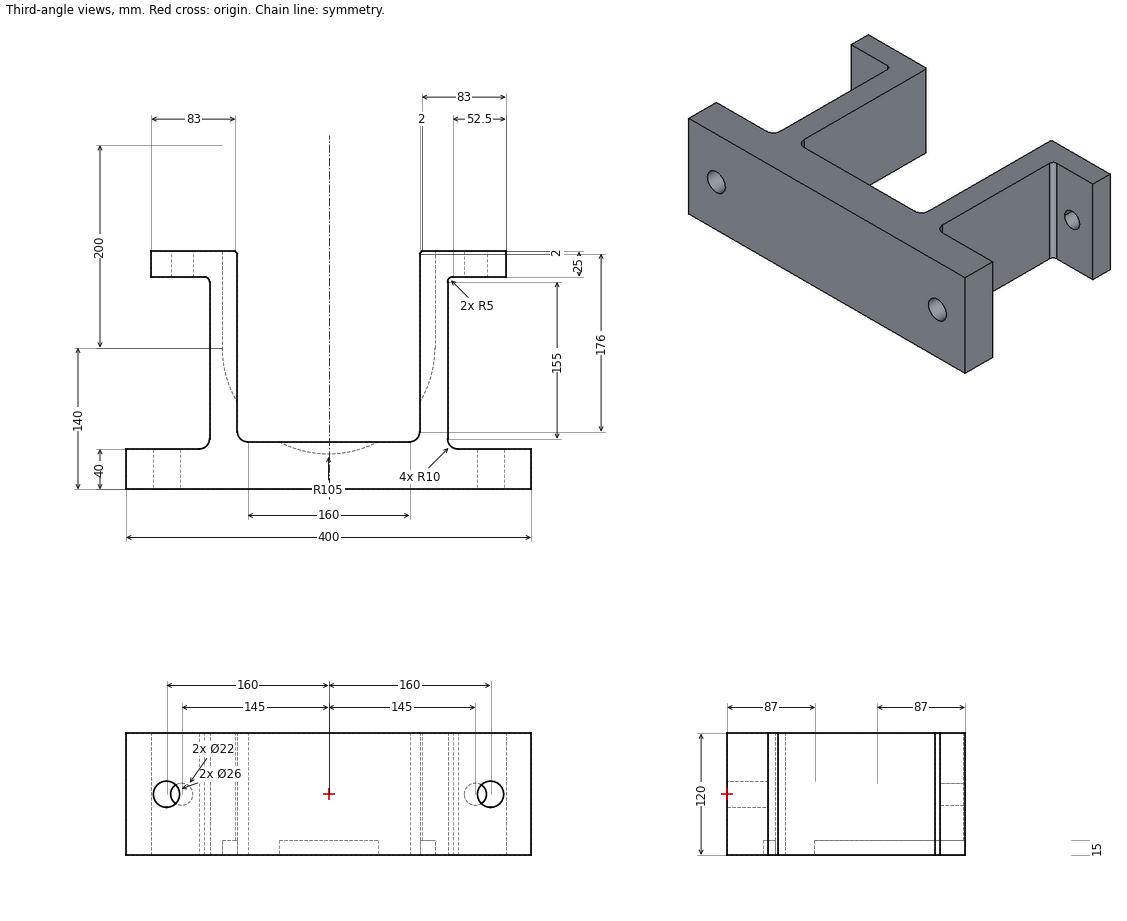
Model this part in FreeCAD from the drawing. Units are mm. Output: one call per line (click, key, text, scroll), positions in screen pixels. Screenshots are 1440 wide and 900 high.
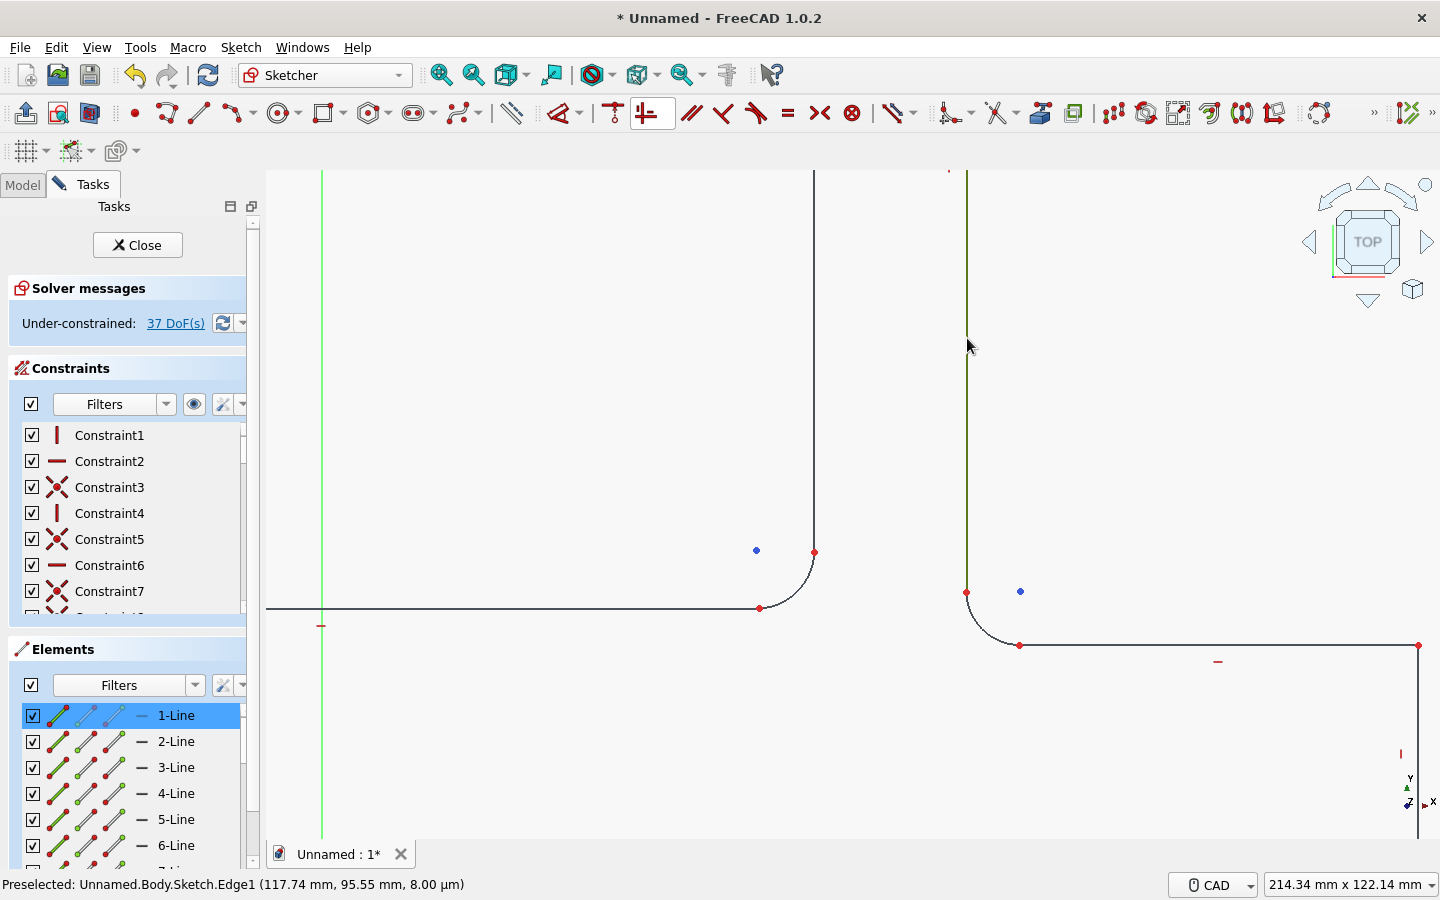
scroll(984, 628, down, 6)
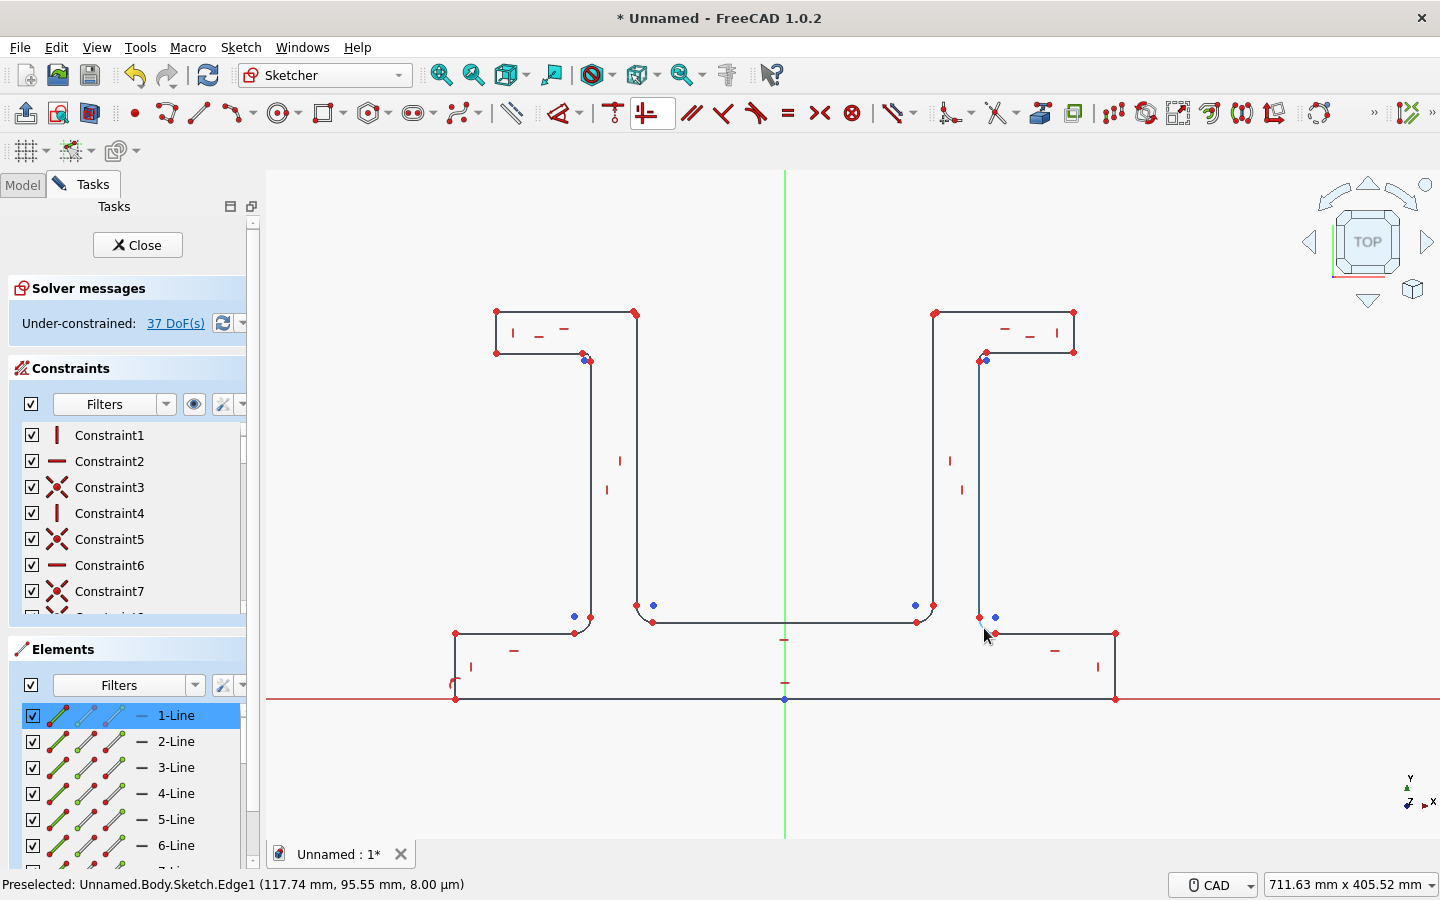
scroll(983, 354, up, 7)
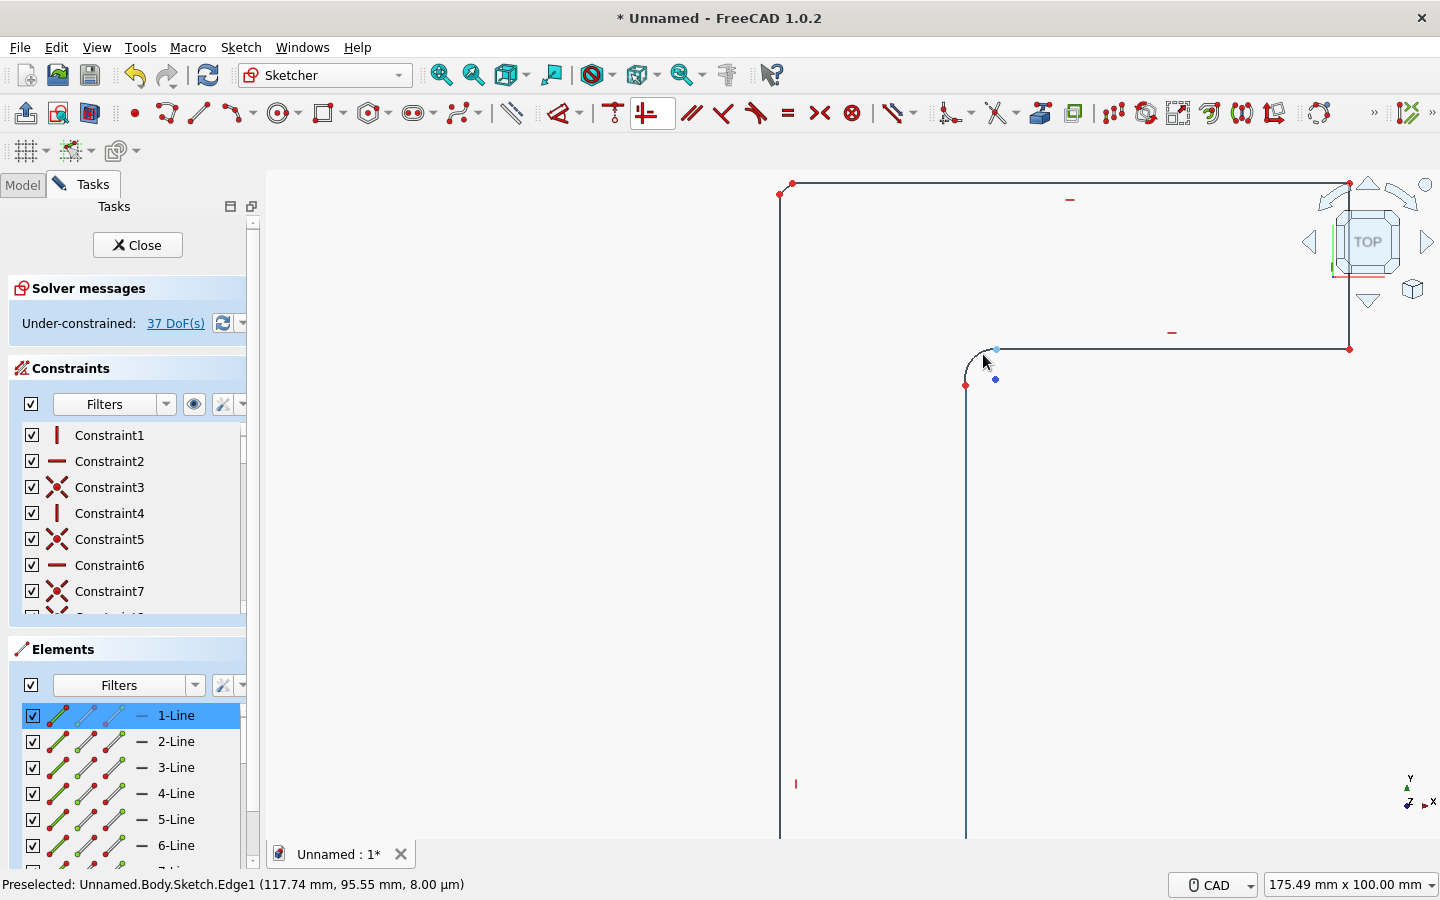
click(980, 353)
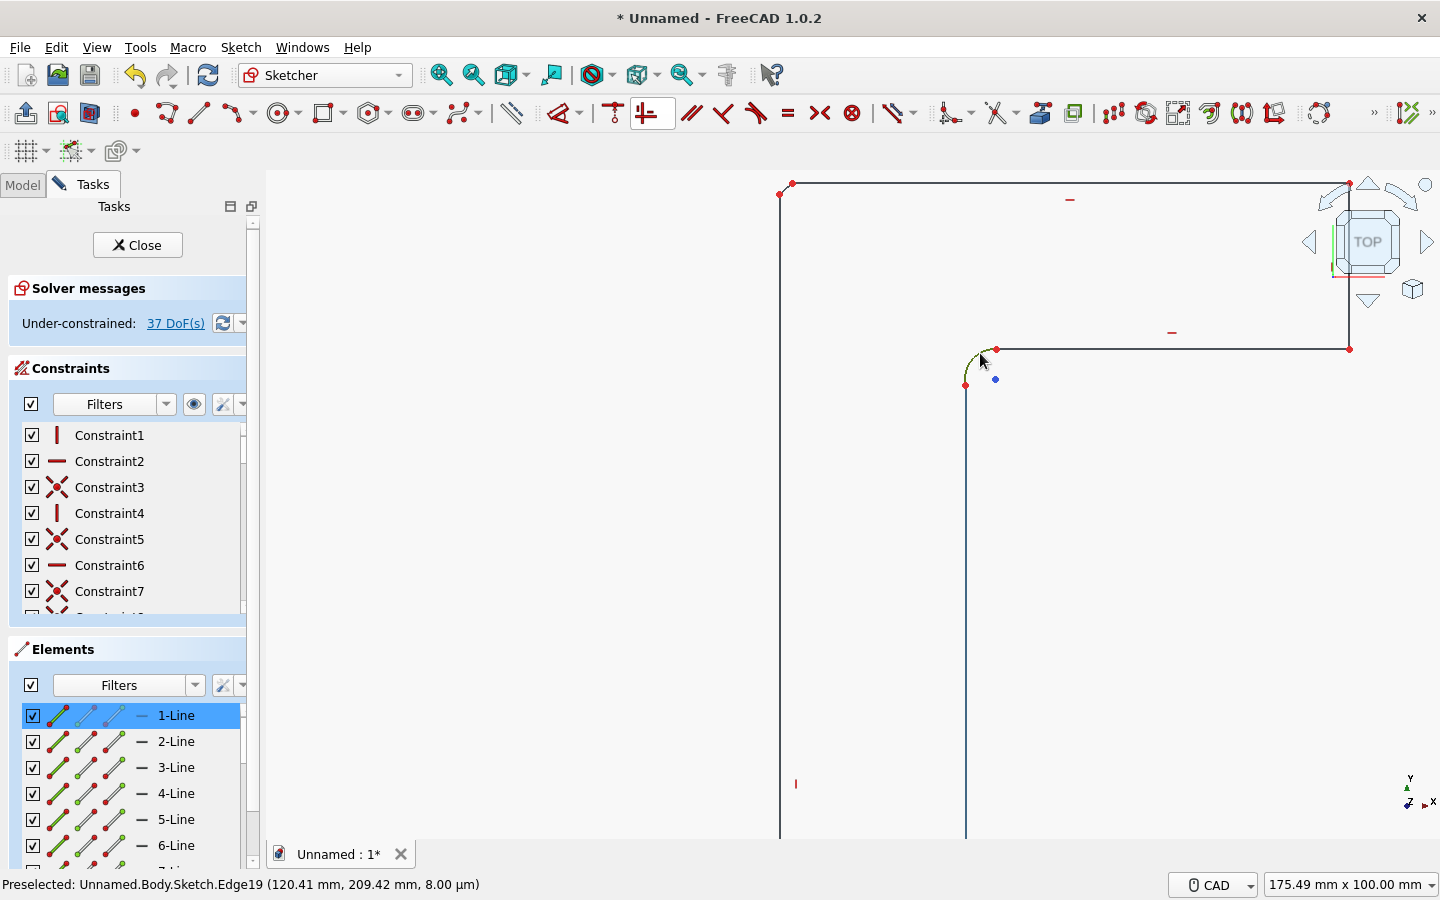
key(t)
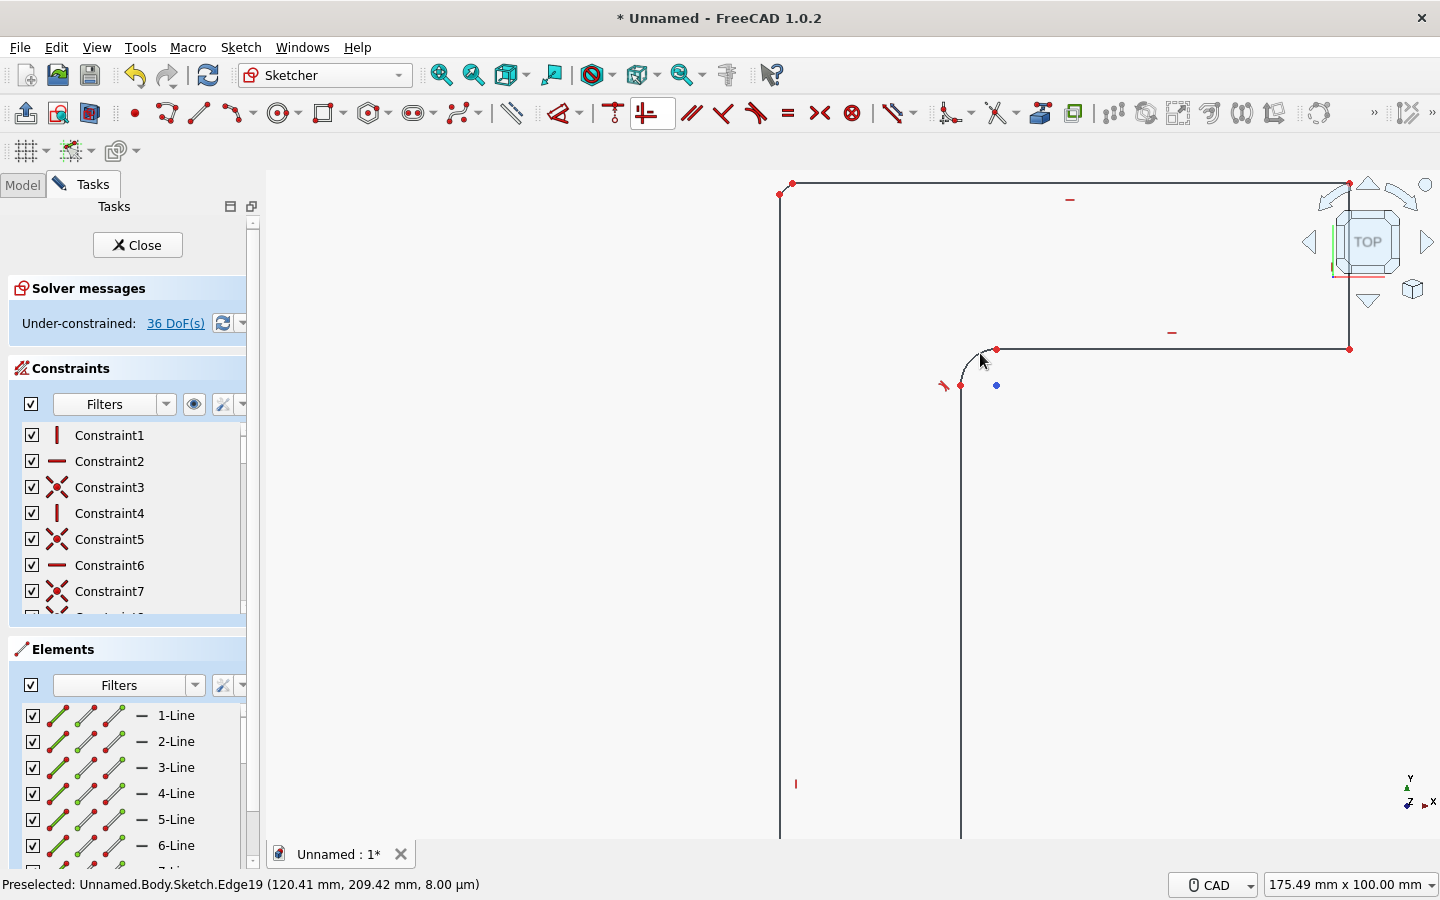
scroll(983, 353, down, 7)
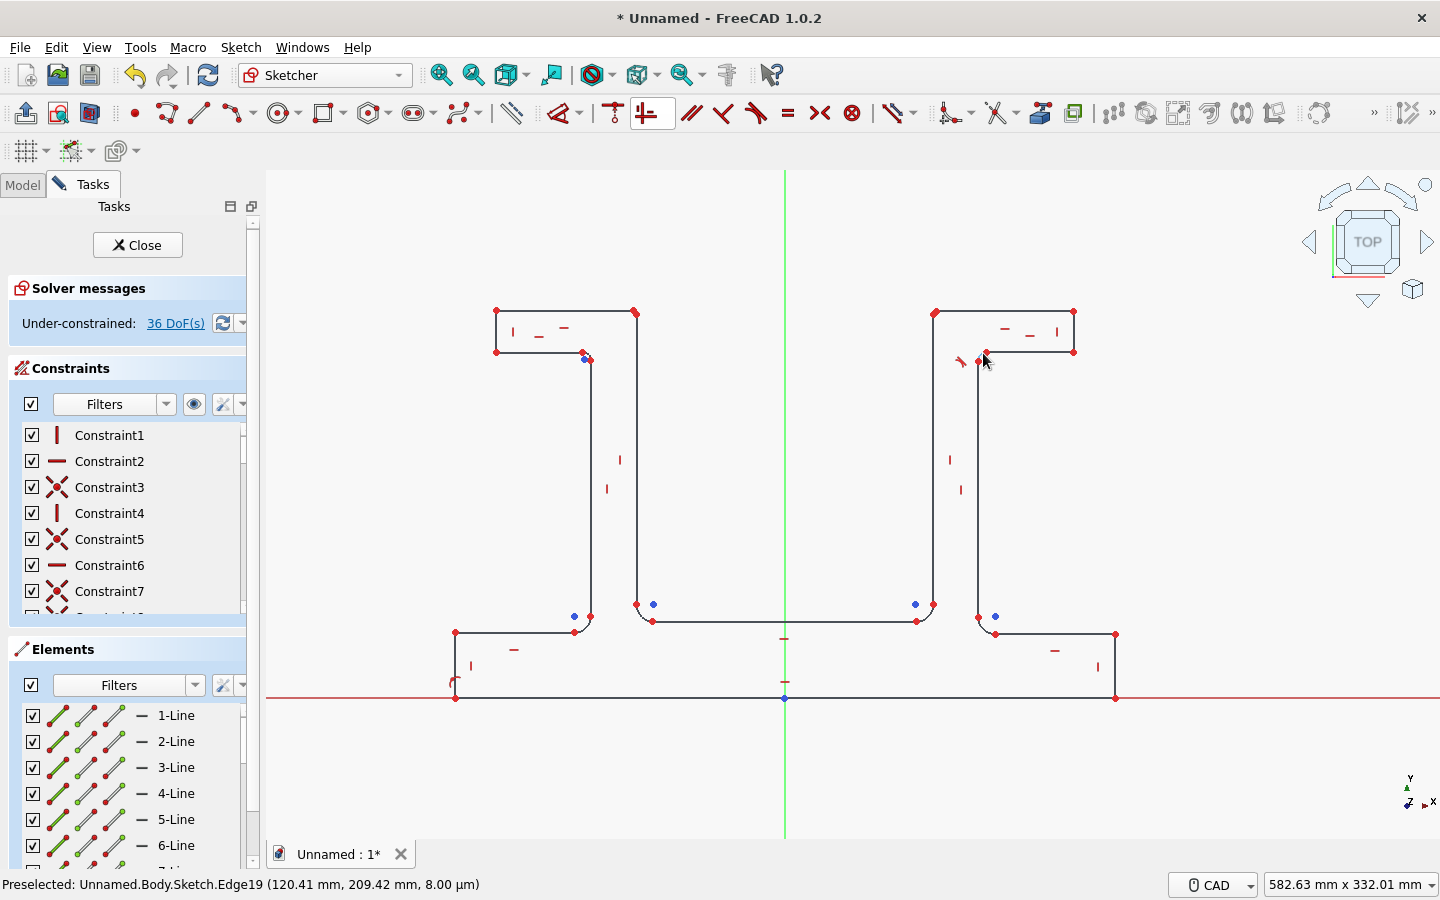
click(978, 438)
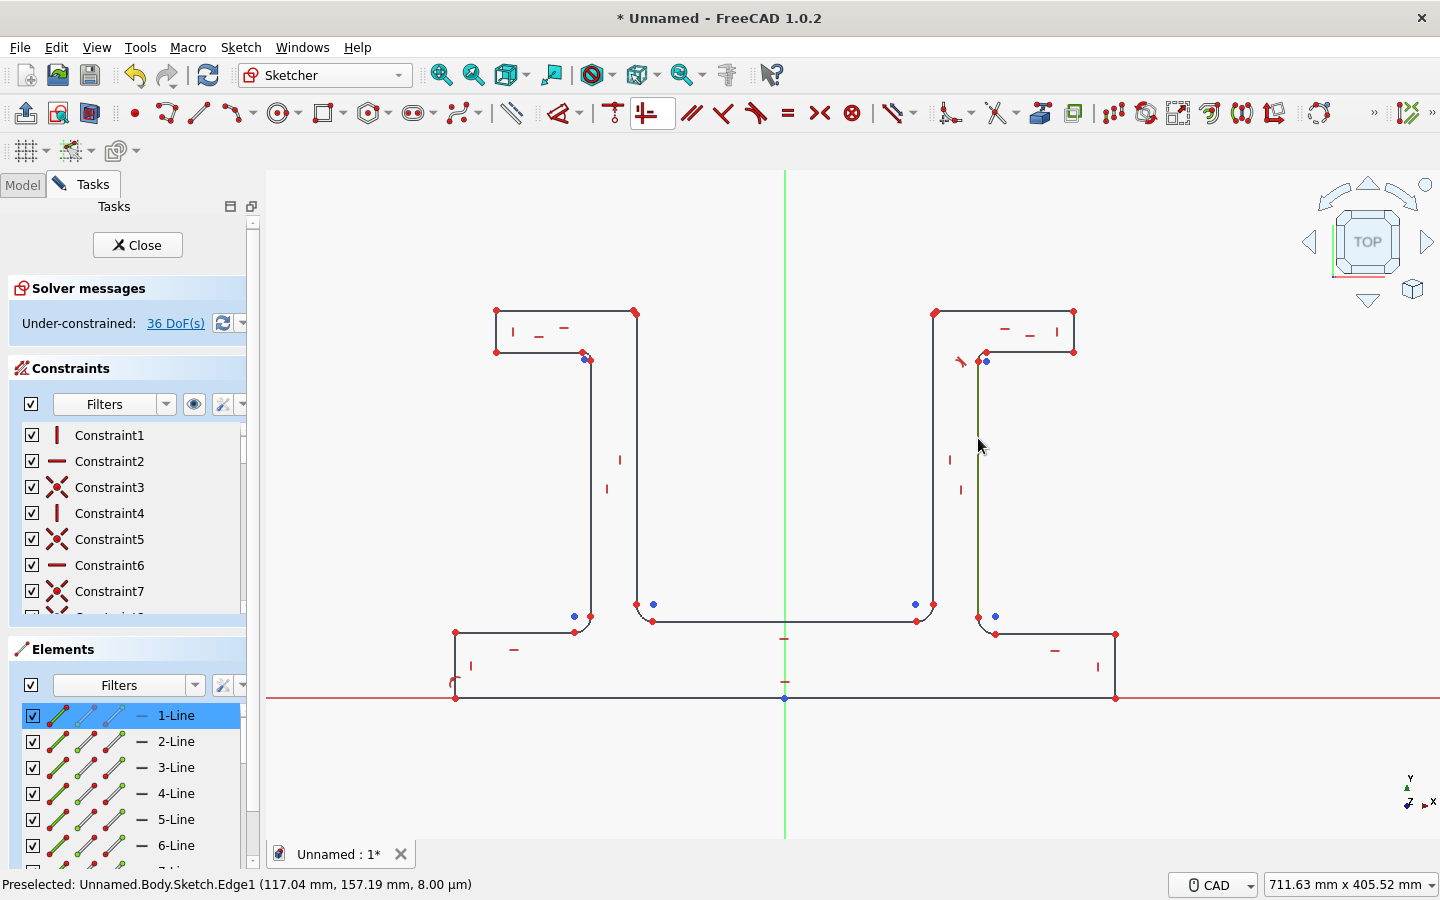
click(983, 629)